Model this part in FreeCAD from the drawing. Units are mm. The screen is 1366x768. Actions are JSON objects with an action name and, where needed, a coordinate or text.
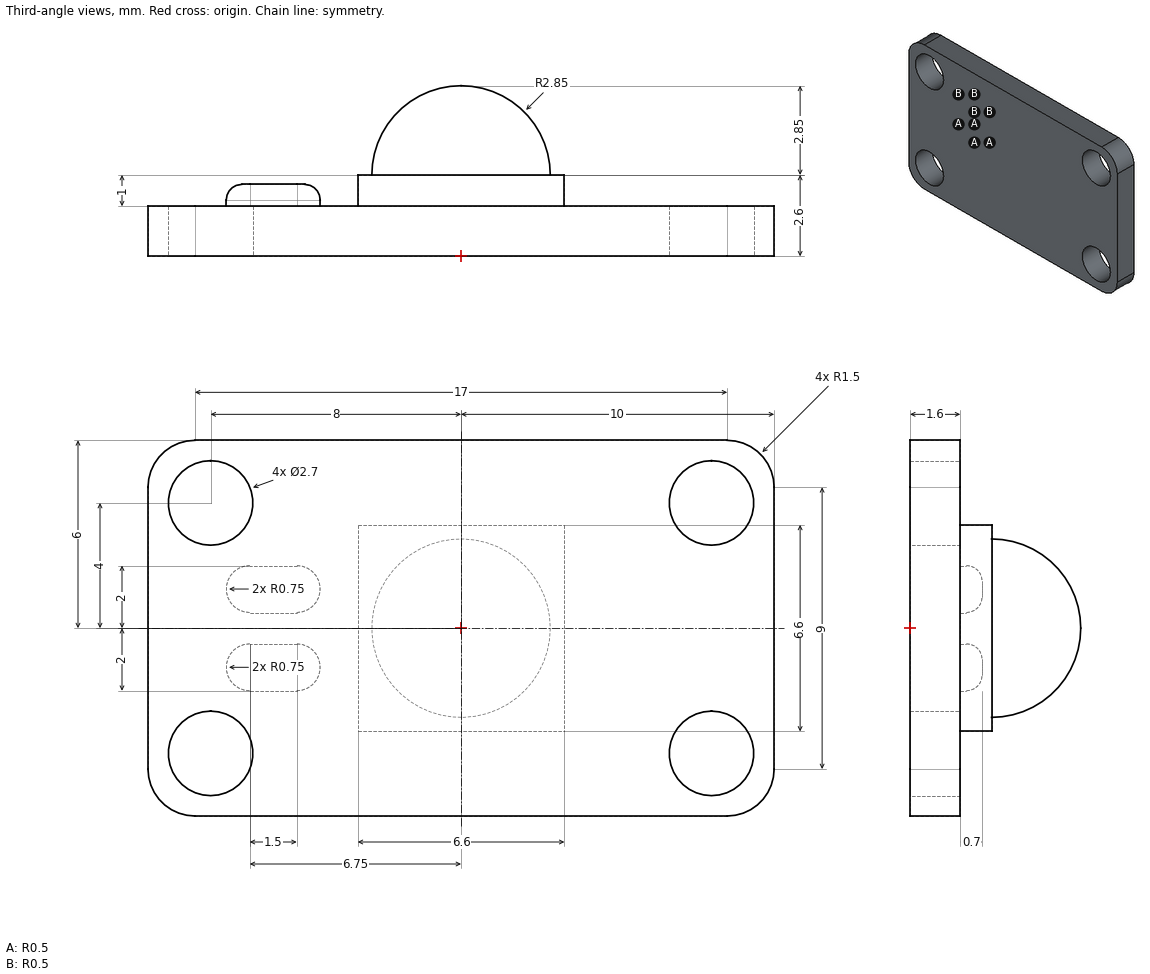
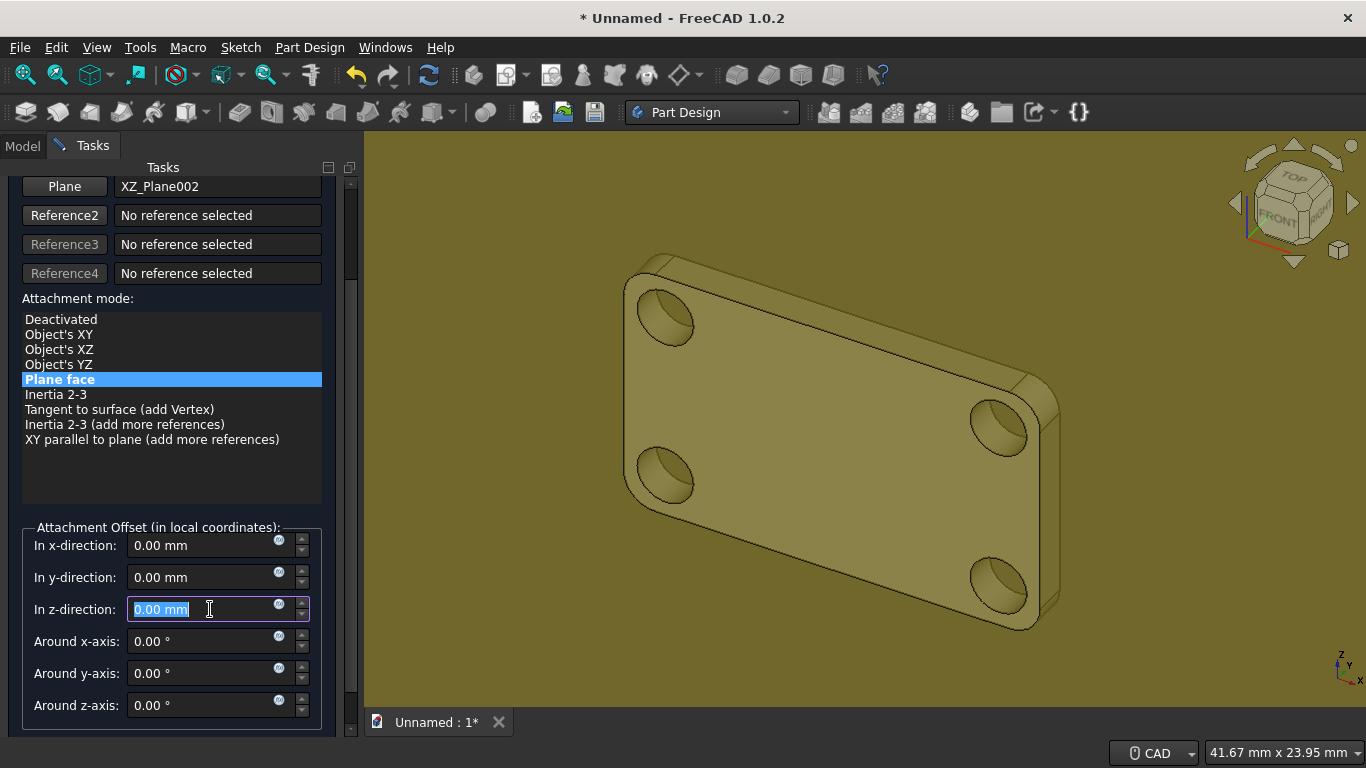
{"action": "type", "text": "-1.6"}
{"action": "key", "text": "Tab"}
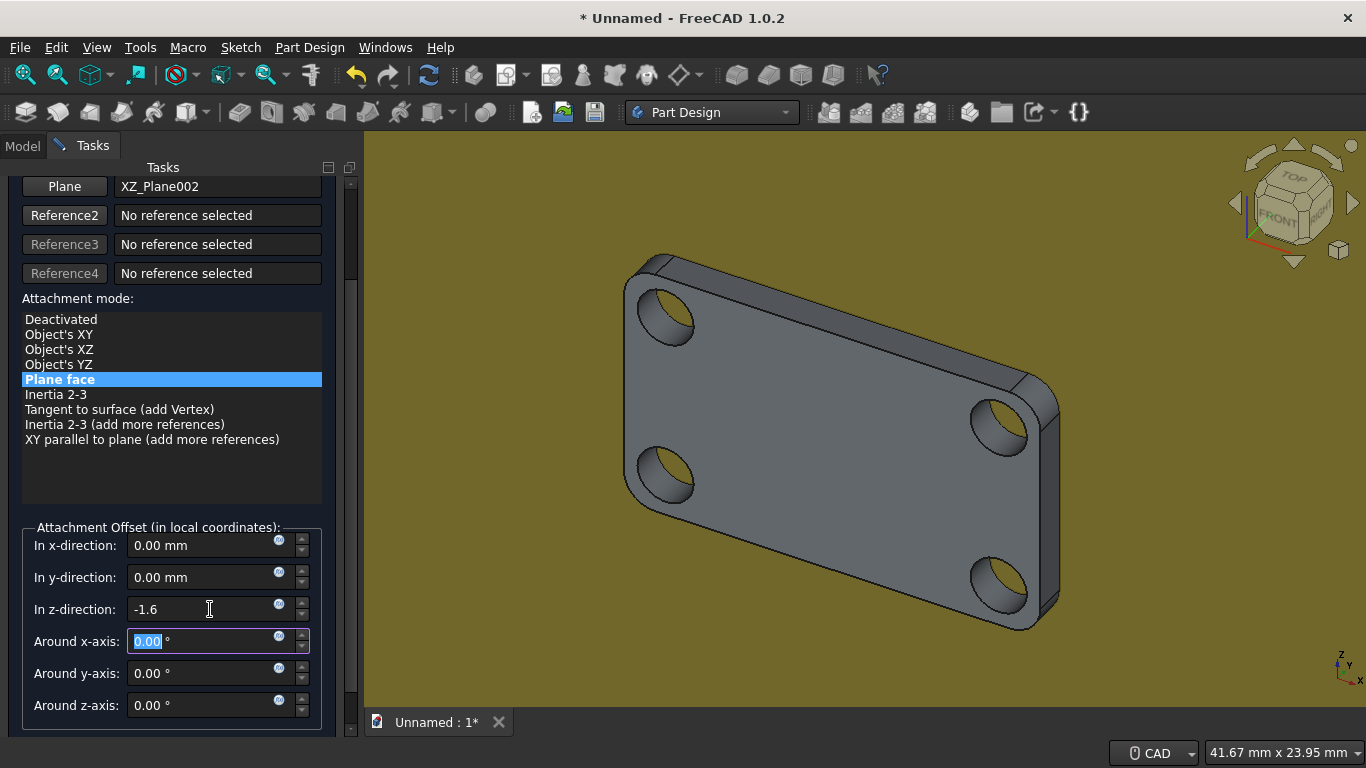
{"action": "scroll", "coordinate": [351, 456], "scroll_direction": "up", "scroll_amount": 3}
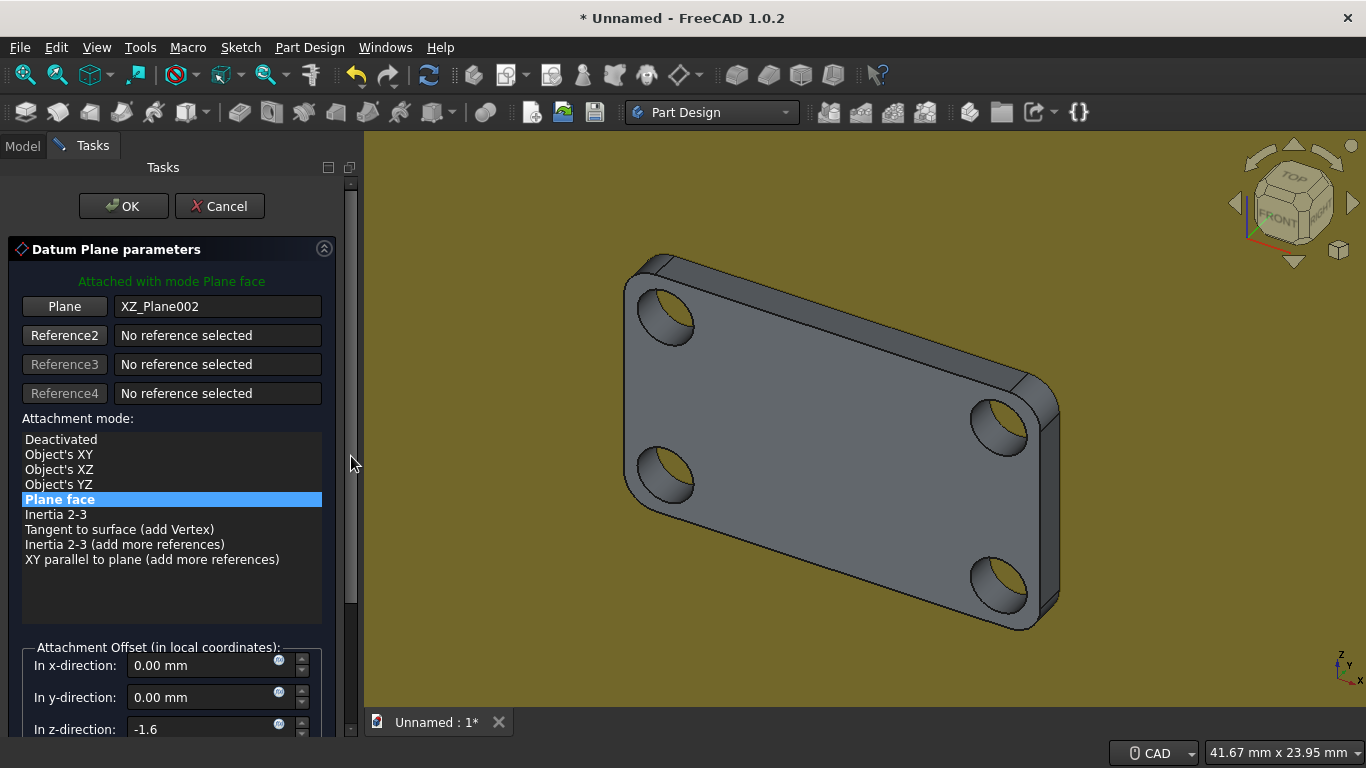
{"action": "left_click", "coordinate": [124, 206]}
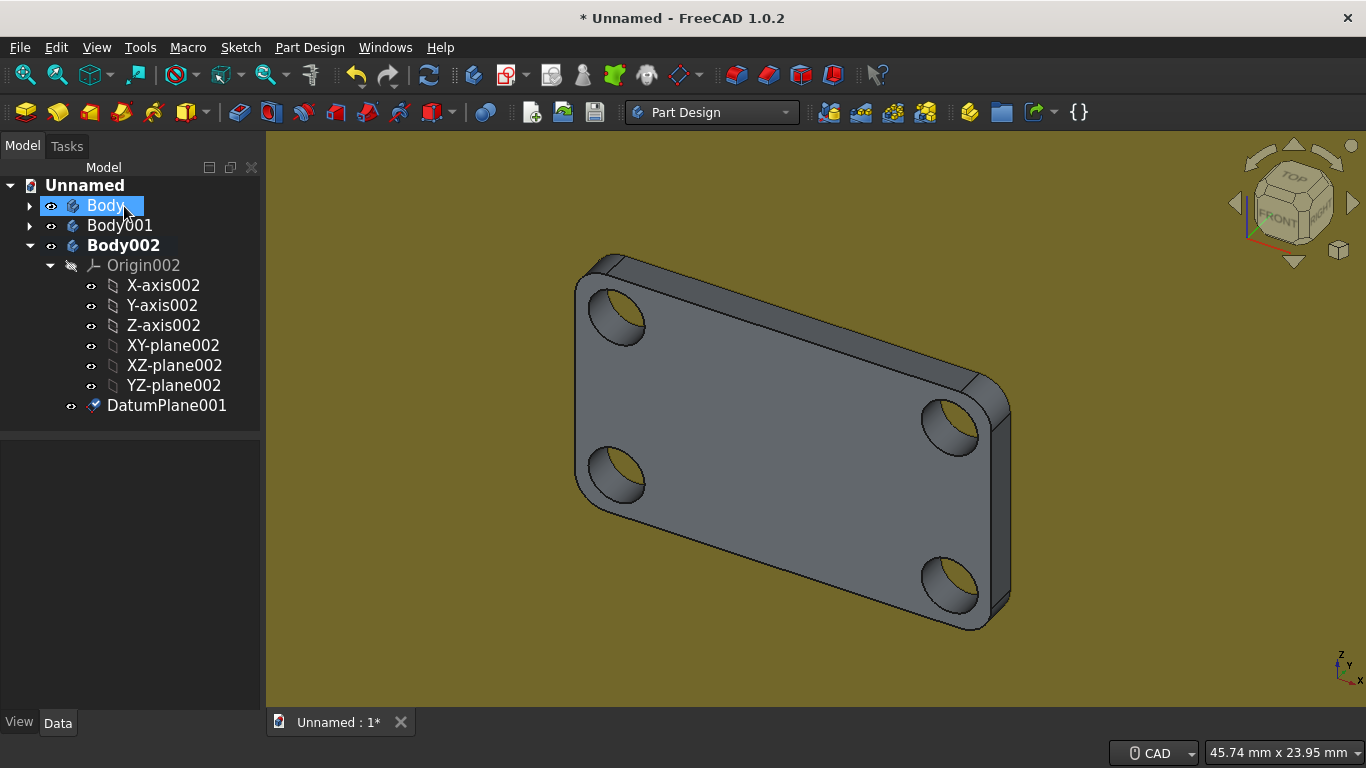
{"action": "left_click", "coordinate": [116, 406]}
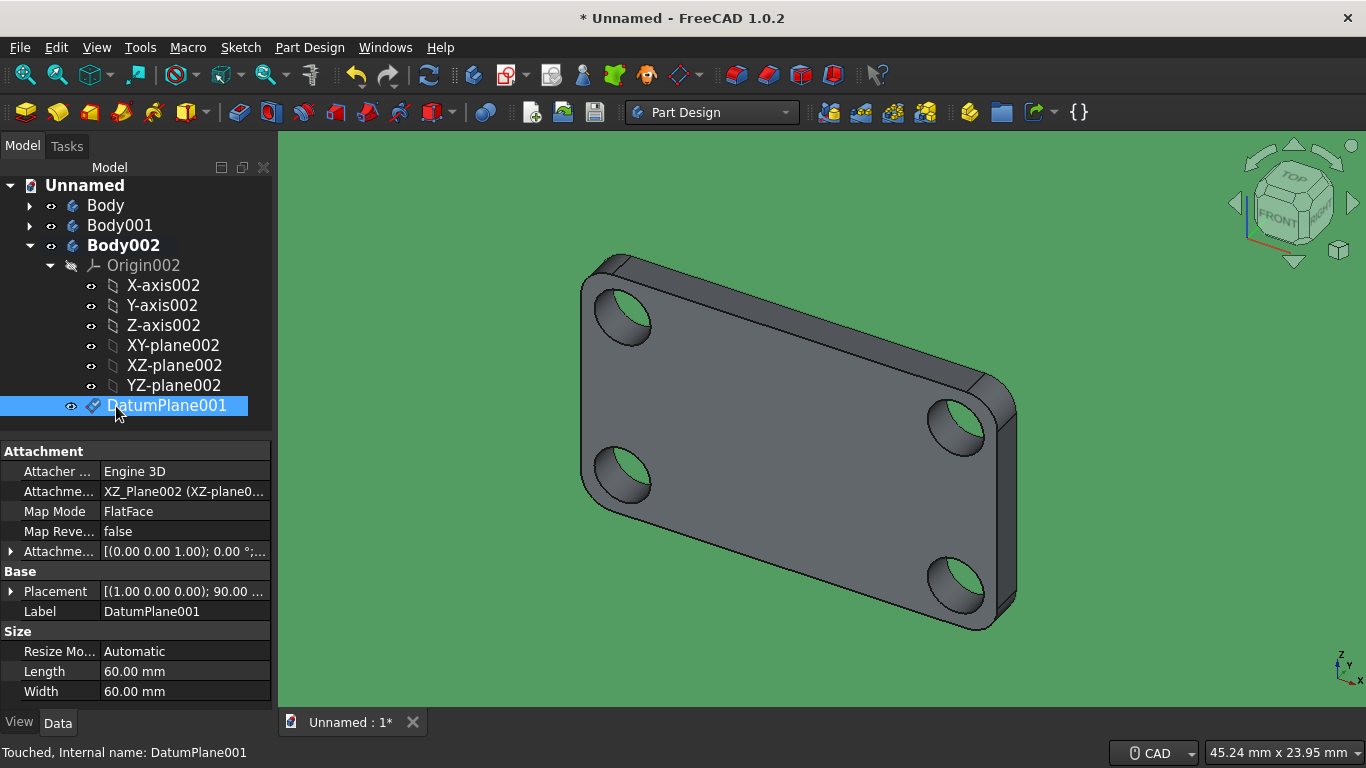
{"action": "left_click", "coordinate": [506, 76]}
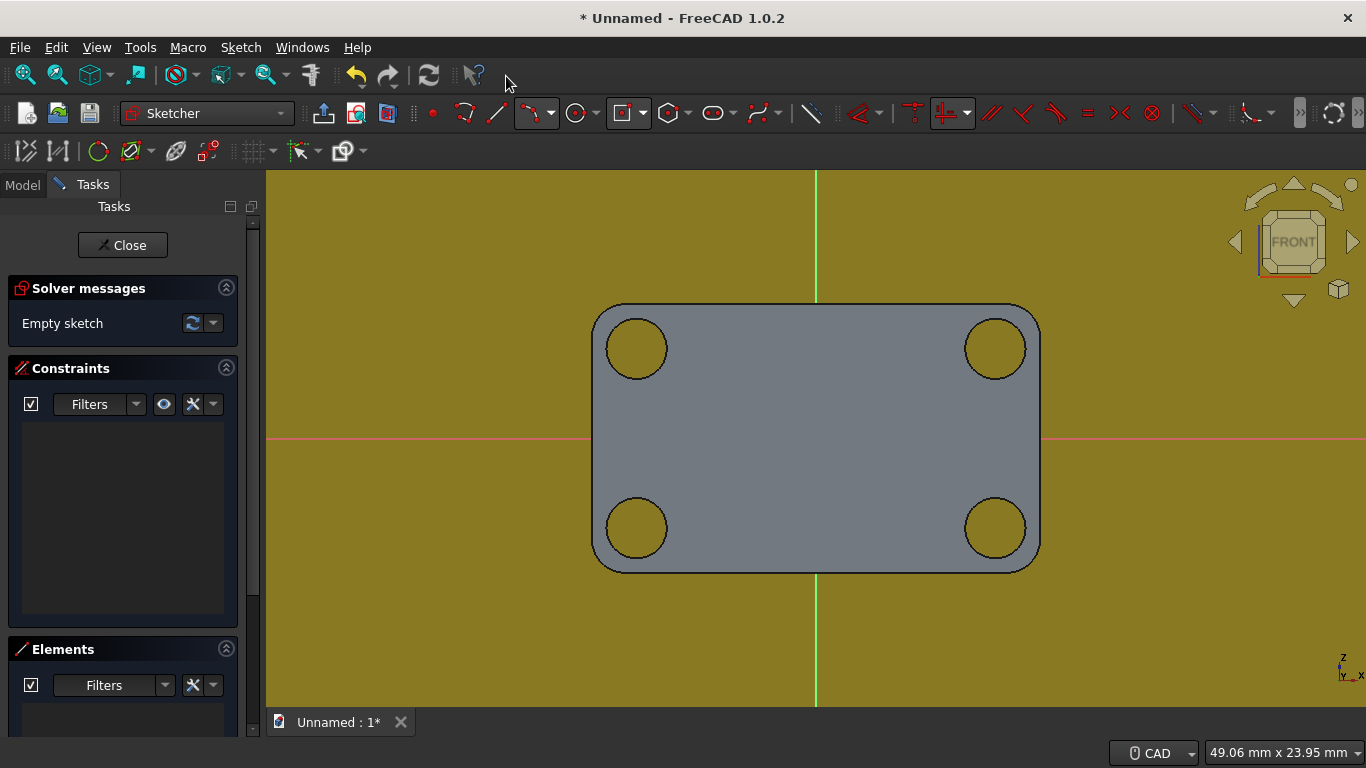
{"action": "scroll", "coordinate": [673, 470], "scroll_direction": "up", "scroll_amount": 11}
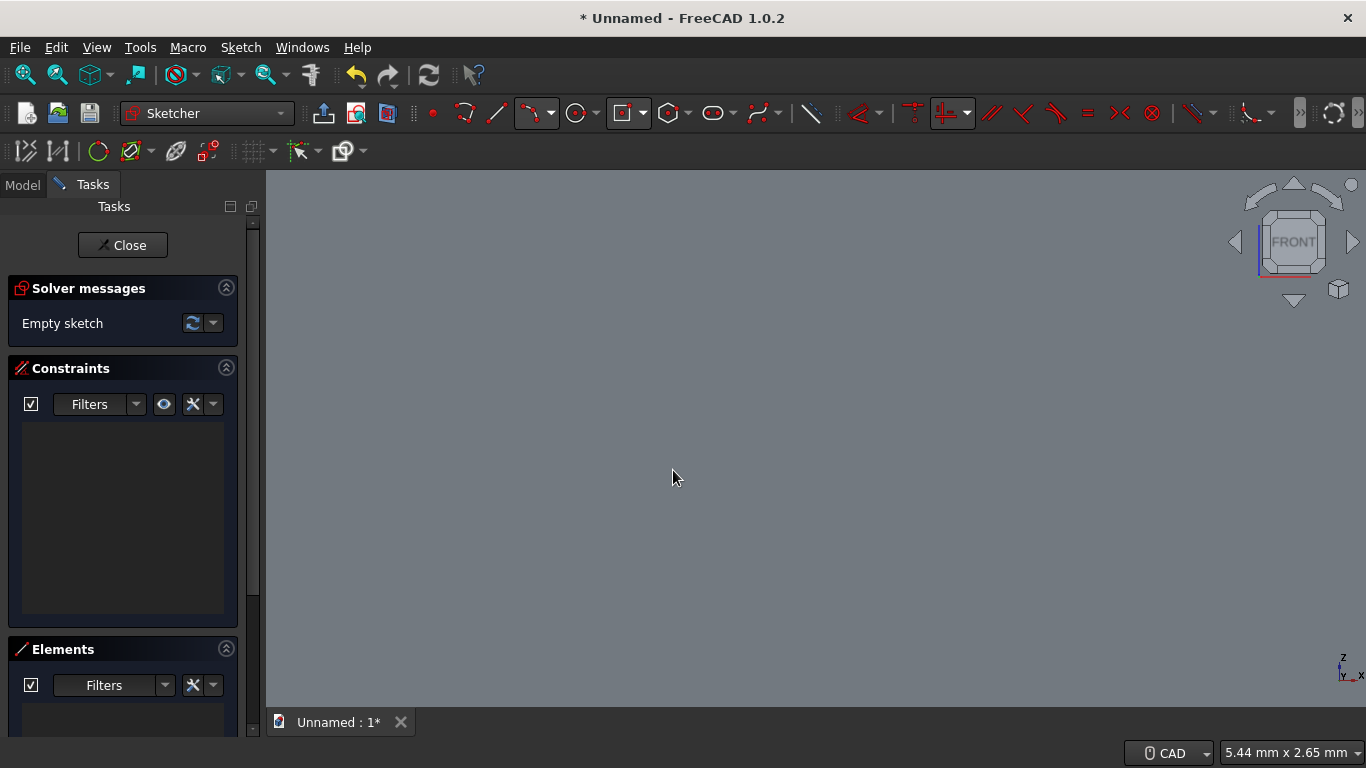
{"action": "left_click", "coordinate": [714, 114]}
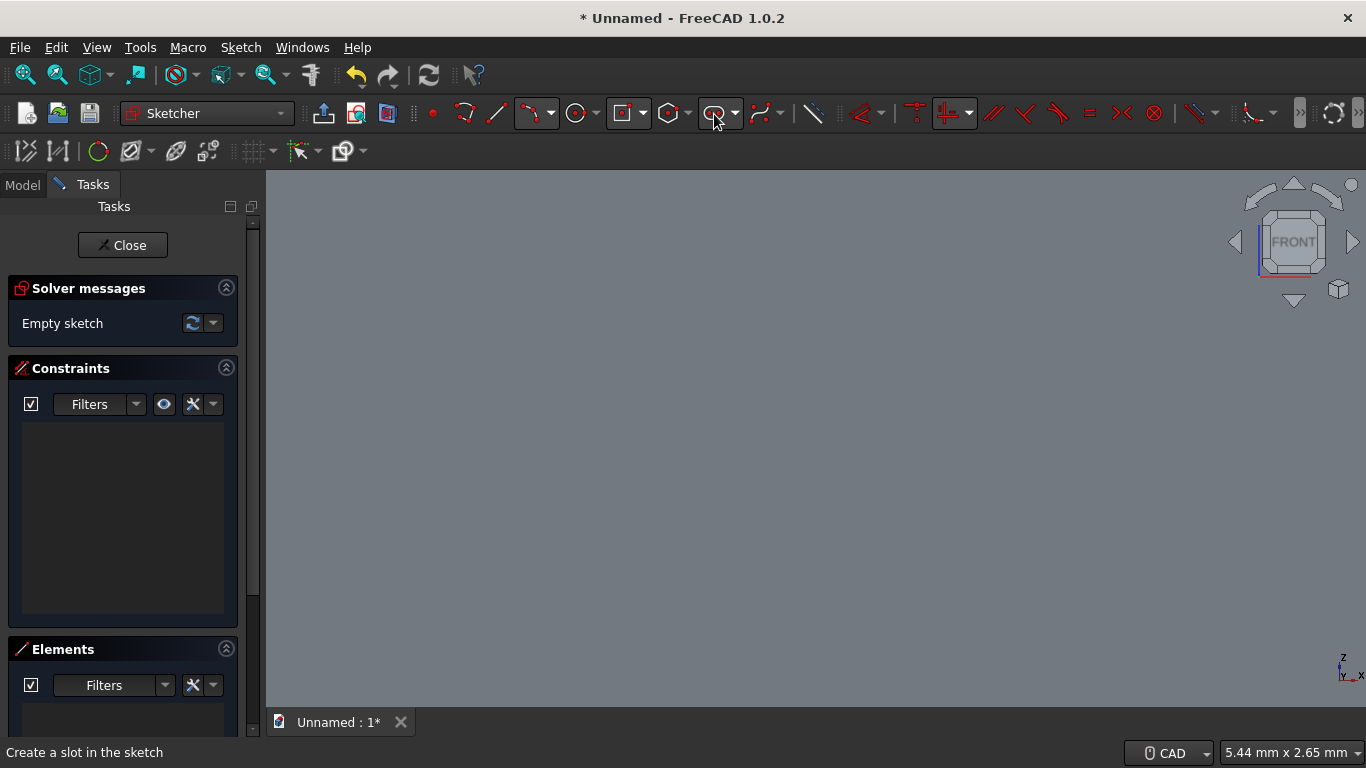
{"action": "left_click", "coordinate": [595, 434]}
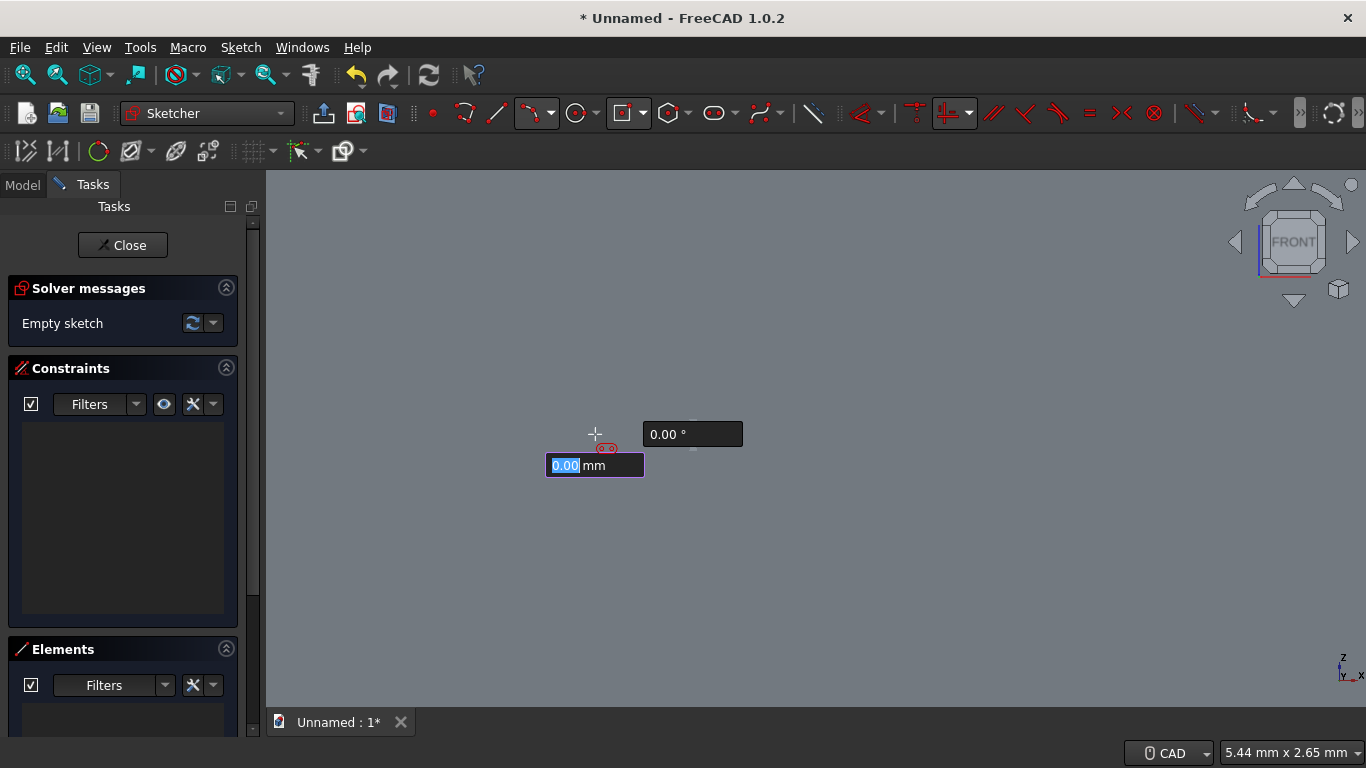
{"action": "left_click", "coordinate": [898, 434]}